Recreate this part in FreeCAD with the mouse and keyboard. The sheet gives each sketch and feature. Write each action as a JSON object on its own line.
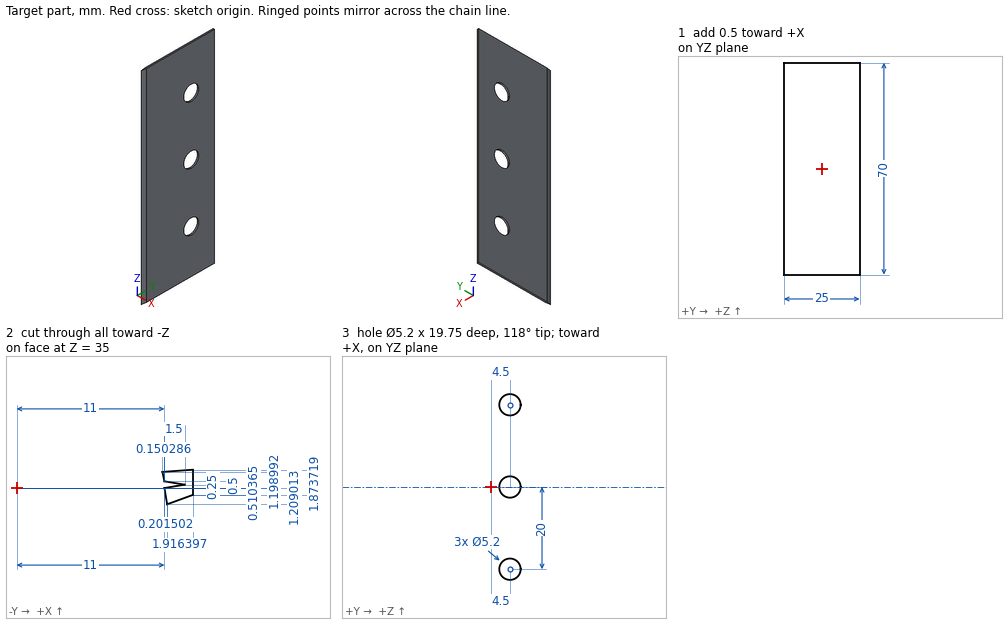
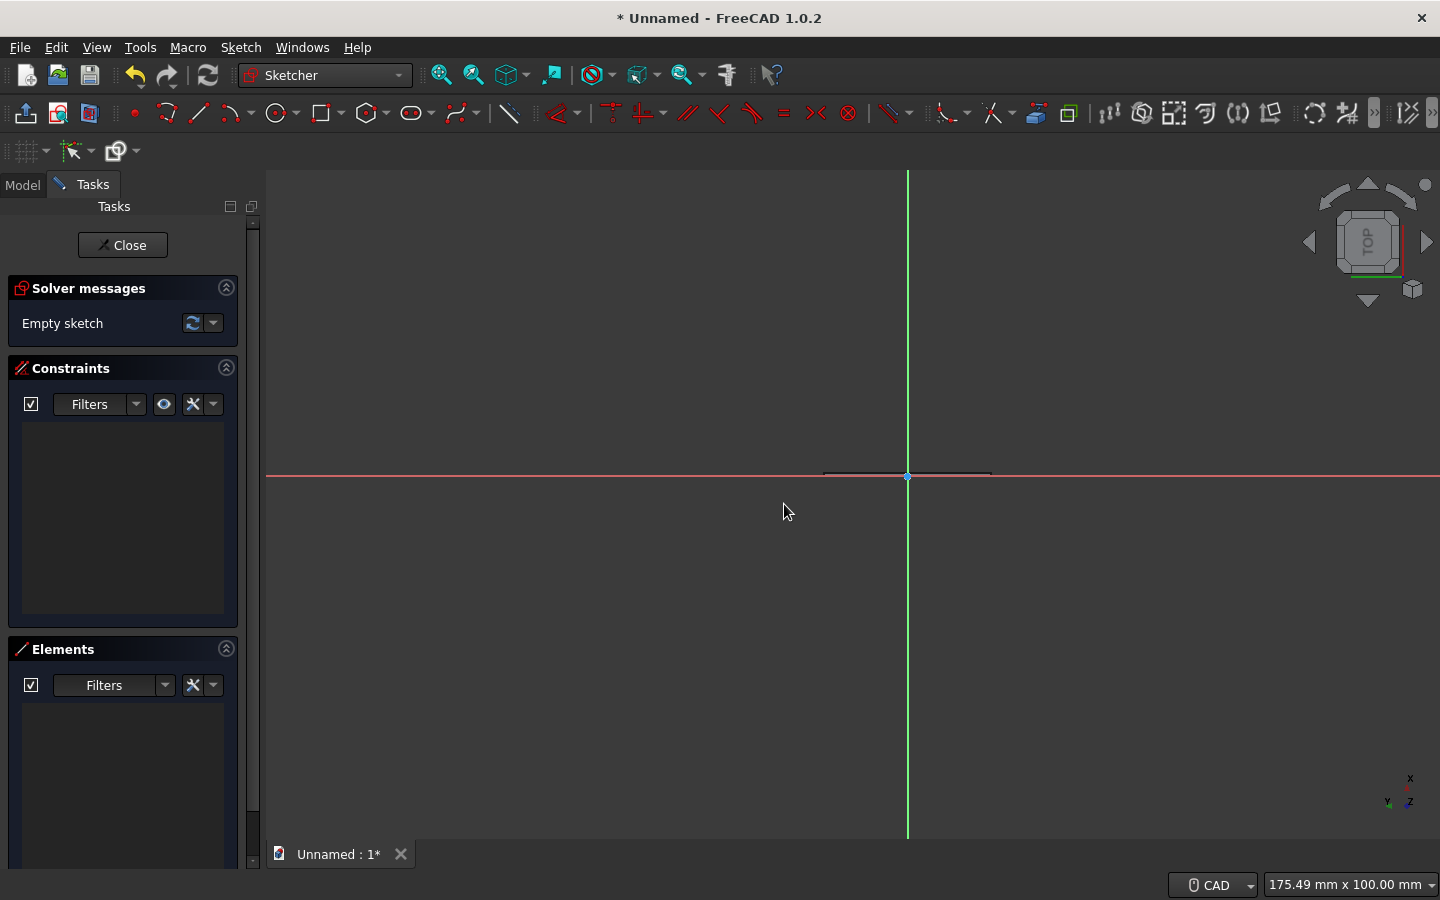
{"action": "scroll", "coordinate": [998, 474], "scroll_direction": "up", "scroll_amount": 15}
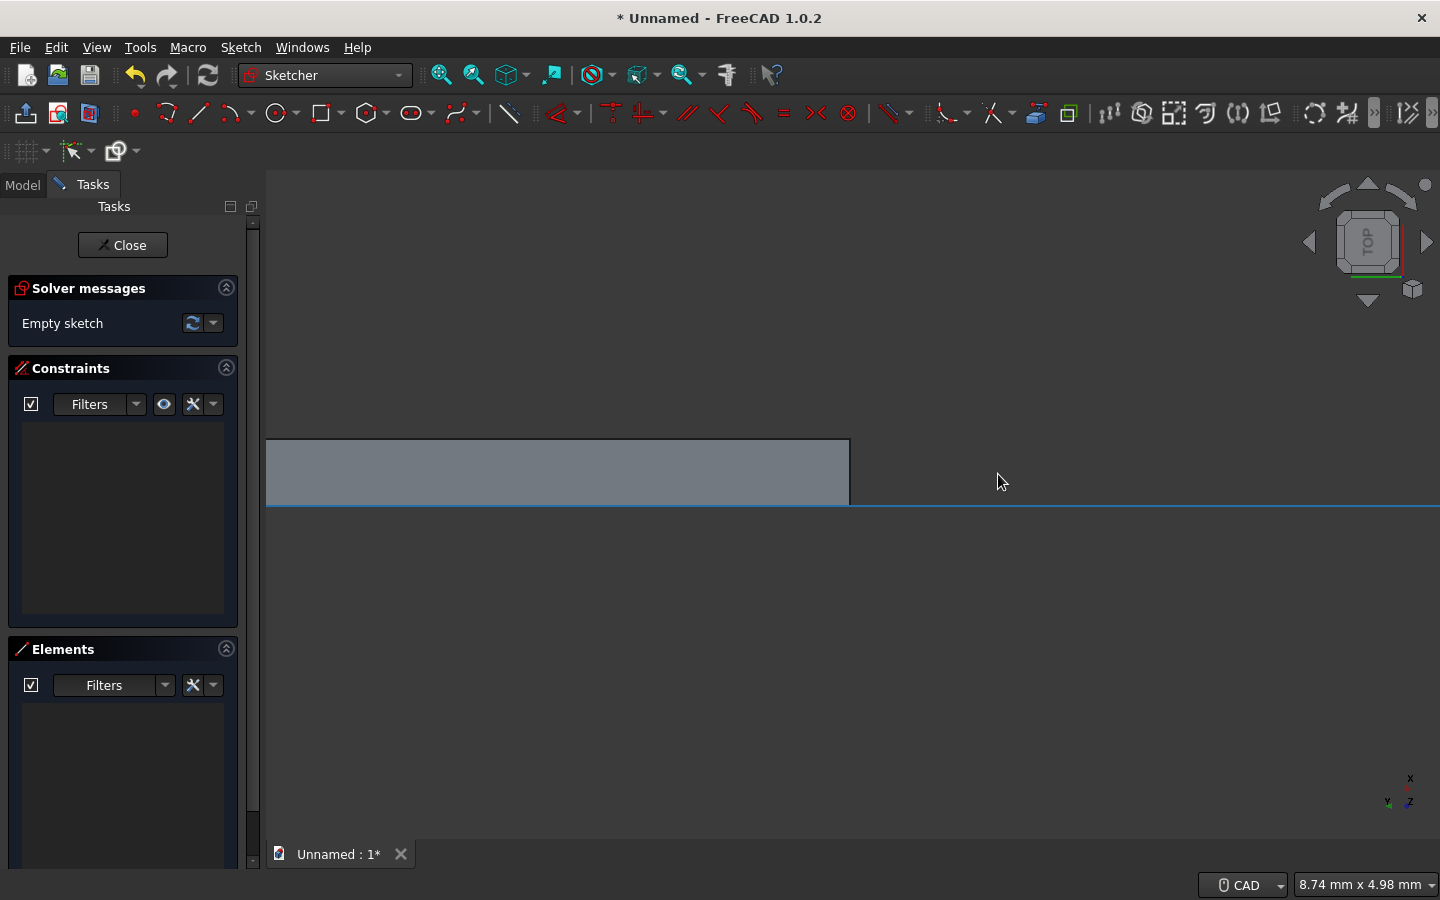
{"action": "left_click", "coordinate": [168, 114]}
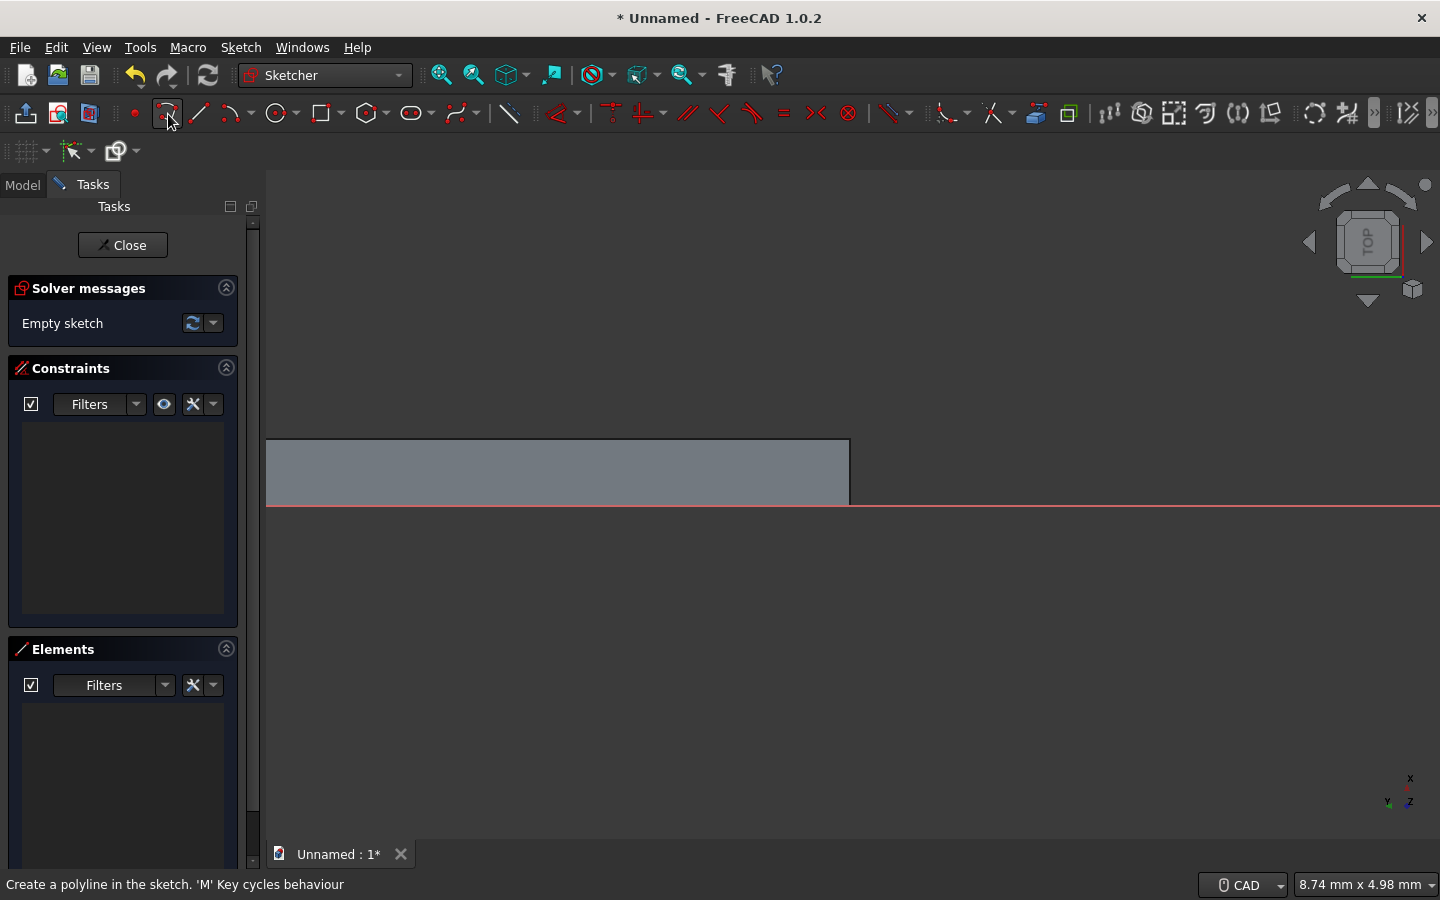
{"action": "left_click", "coordinate": [629, 345]}
{"action": "left_click", "coordinate": [649, 439]}
{"action": "left_click", "coordinate": [850, 473]}
{"action": "left_click", "coordinate": [649, 506]}
{"action": "left_click", "coordinate": [676, 669]}
{"action": "left_click", "coordinate": [933, 575]}
{"action": "left_click", "coordinate": [933, 323]}
{"action": "left_click", "coordinate": [629, 346]}
{"action": "key", "text": "Escape"}
{"action": "key", "text": "Escape"}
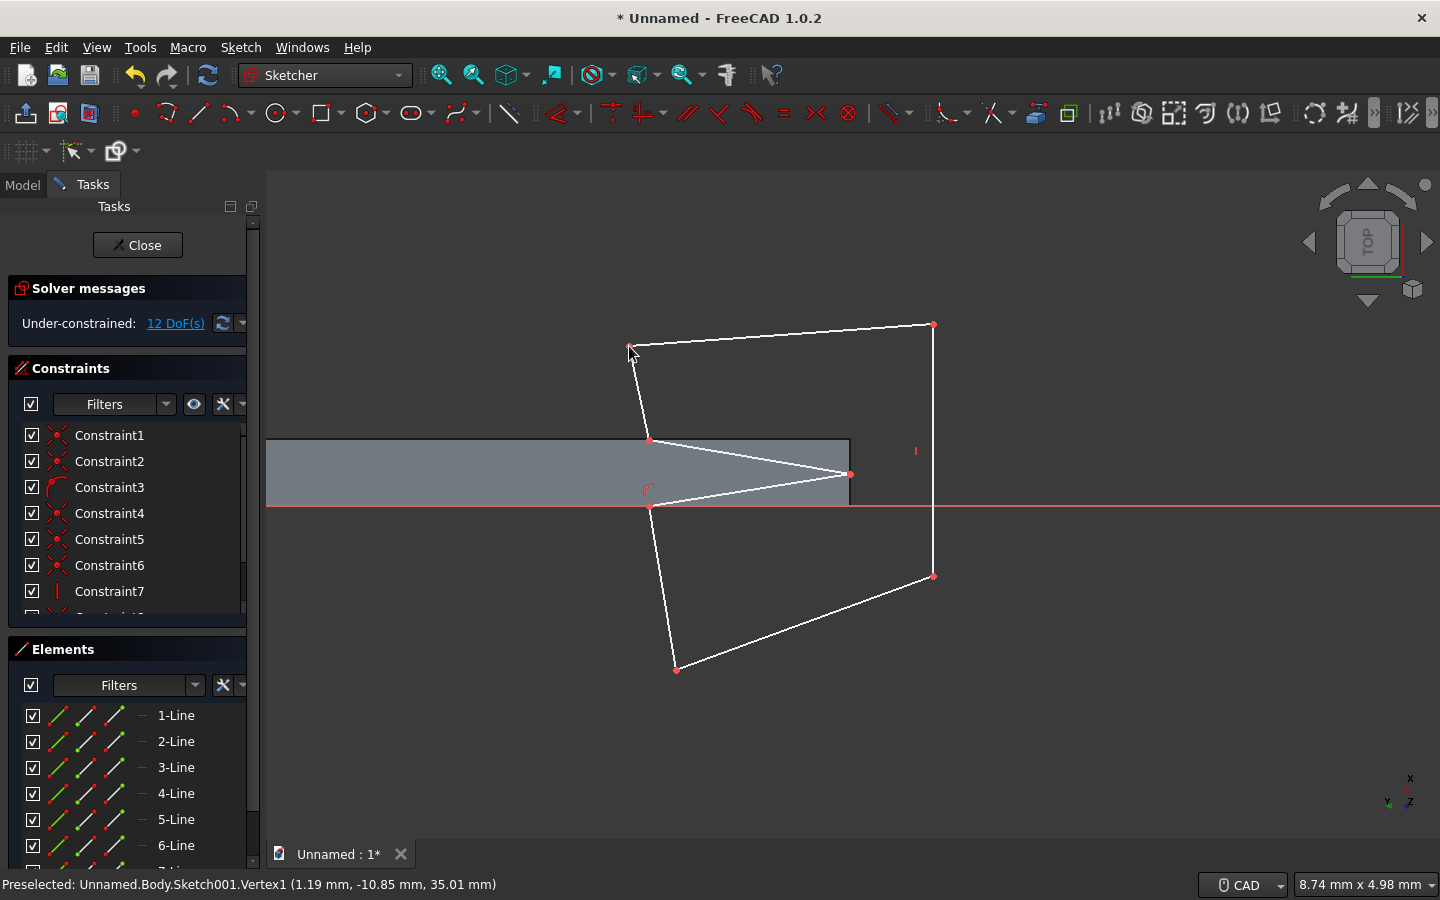
{"action": "key", "text": "d"}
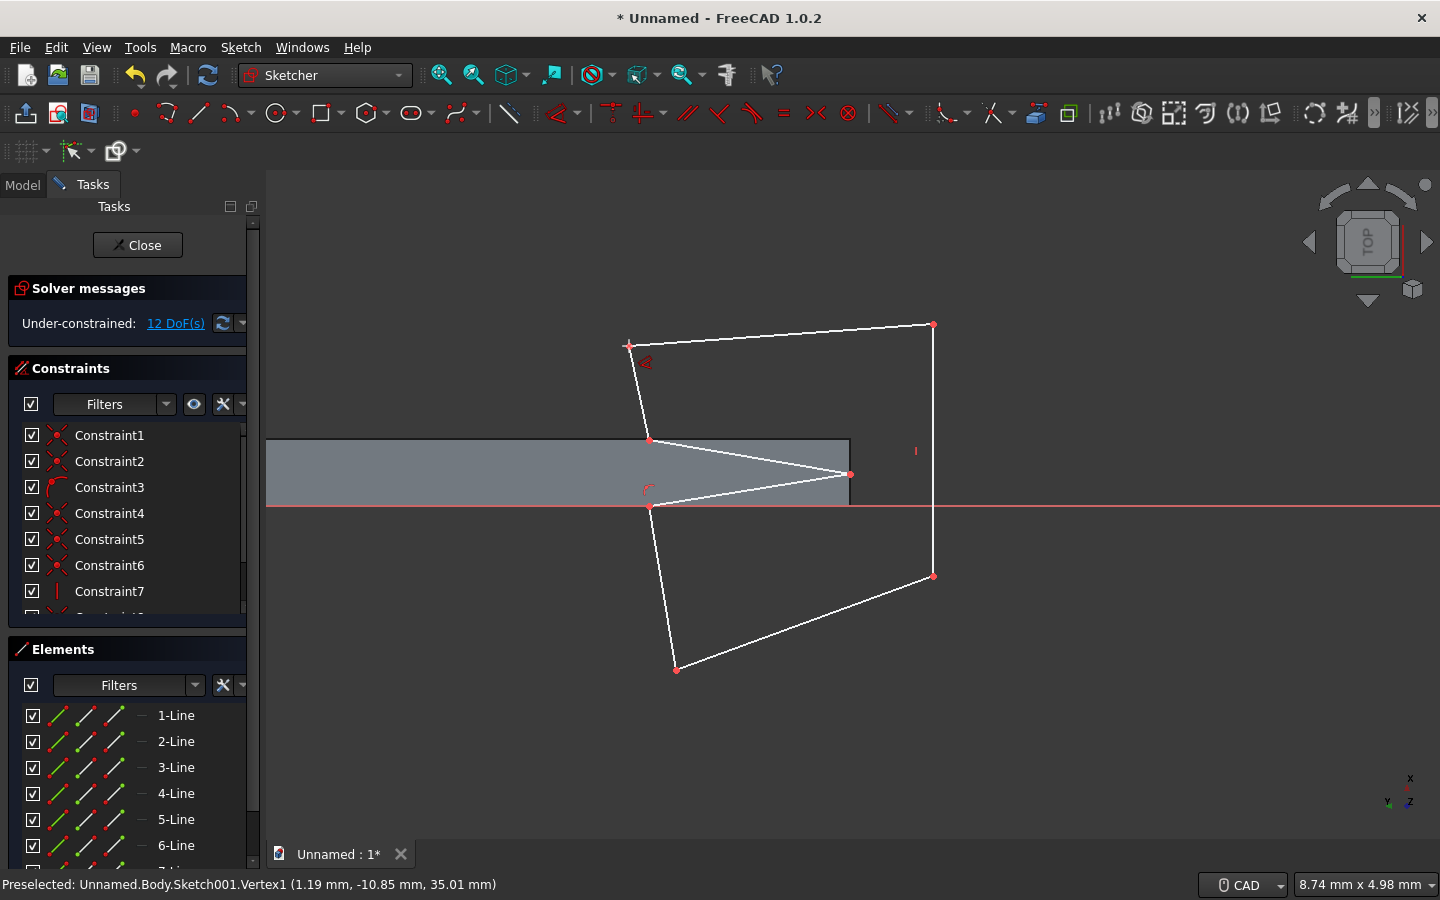
{"action": "left_click", "coordinate": [649, 440]}
{"action": "left_click", "coordinate": [472, 406]}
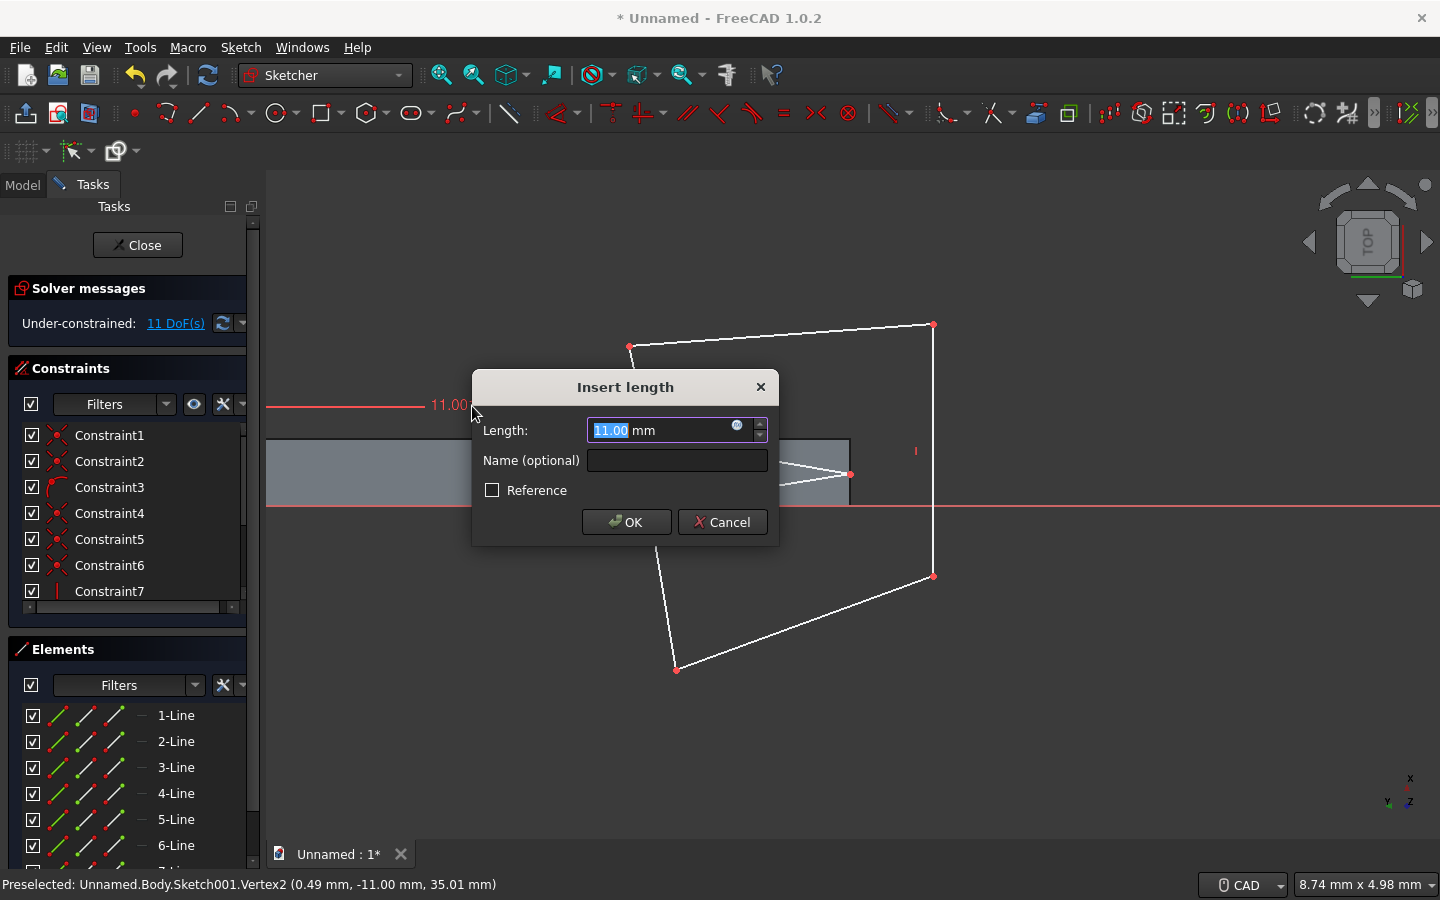
{"action": "type", "text": "11"}
{"action": "key", "text": "Return"}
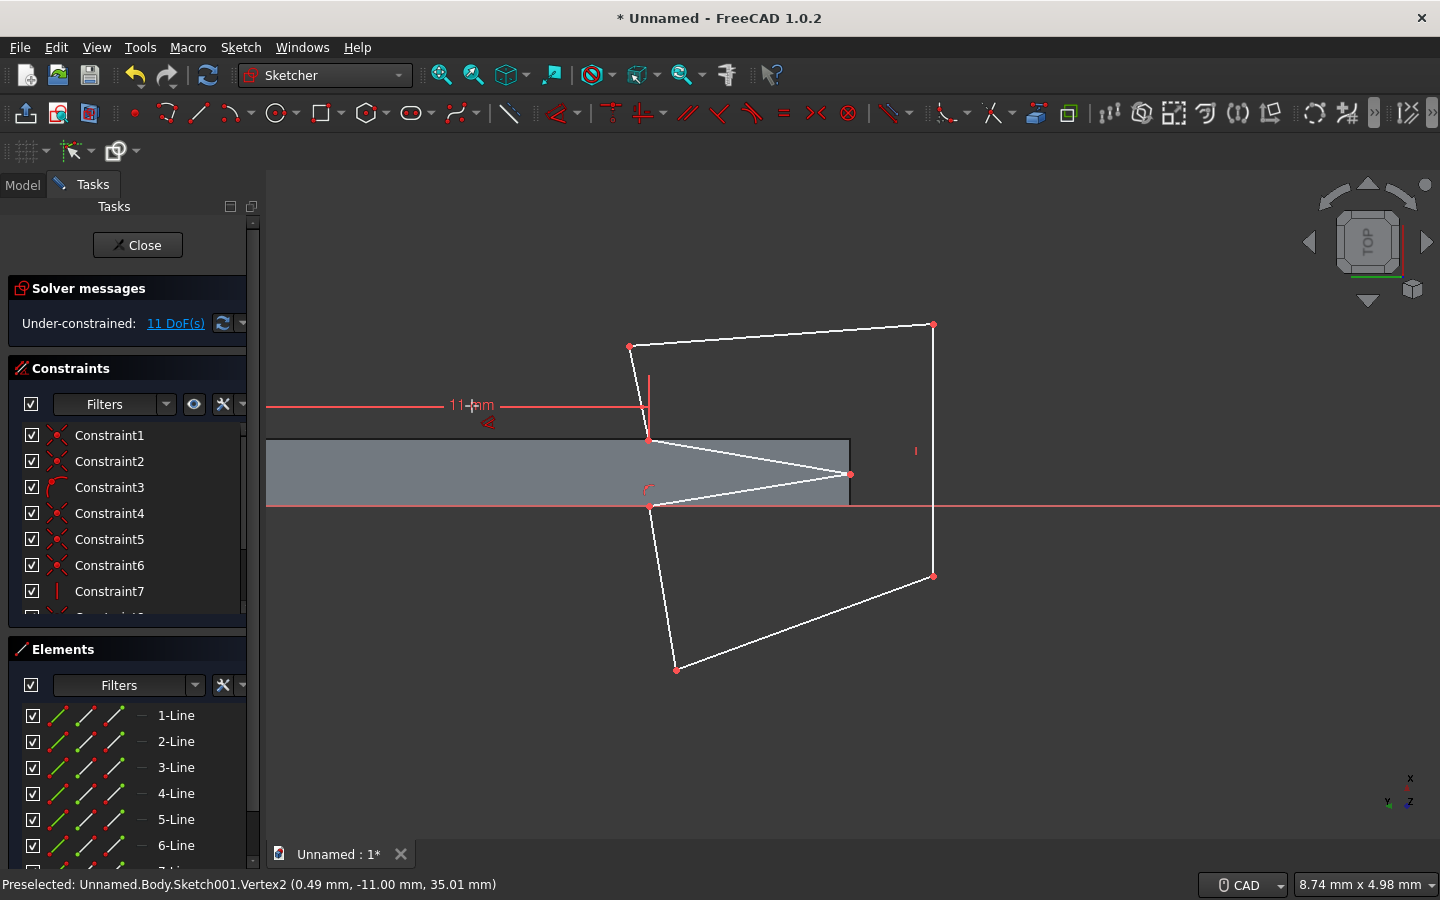
{"action": "left_click", "coordinate": [649, 506]}
{"action": "left_click", "coordinate": [472, 540]}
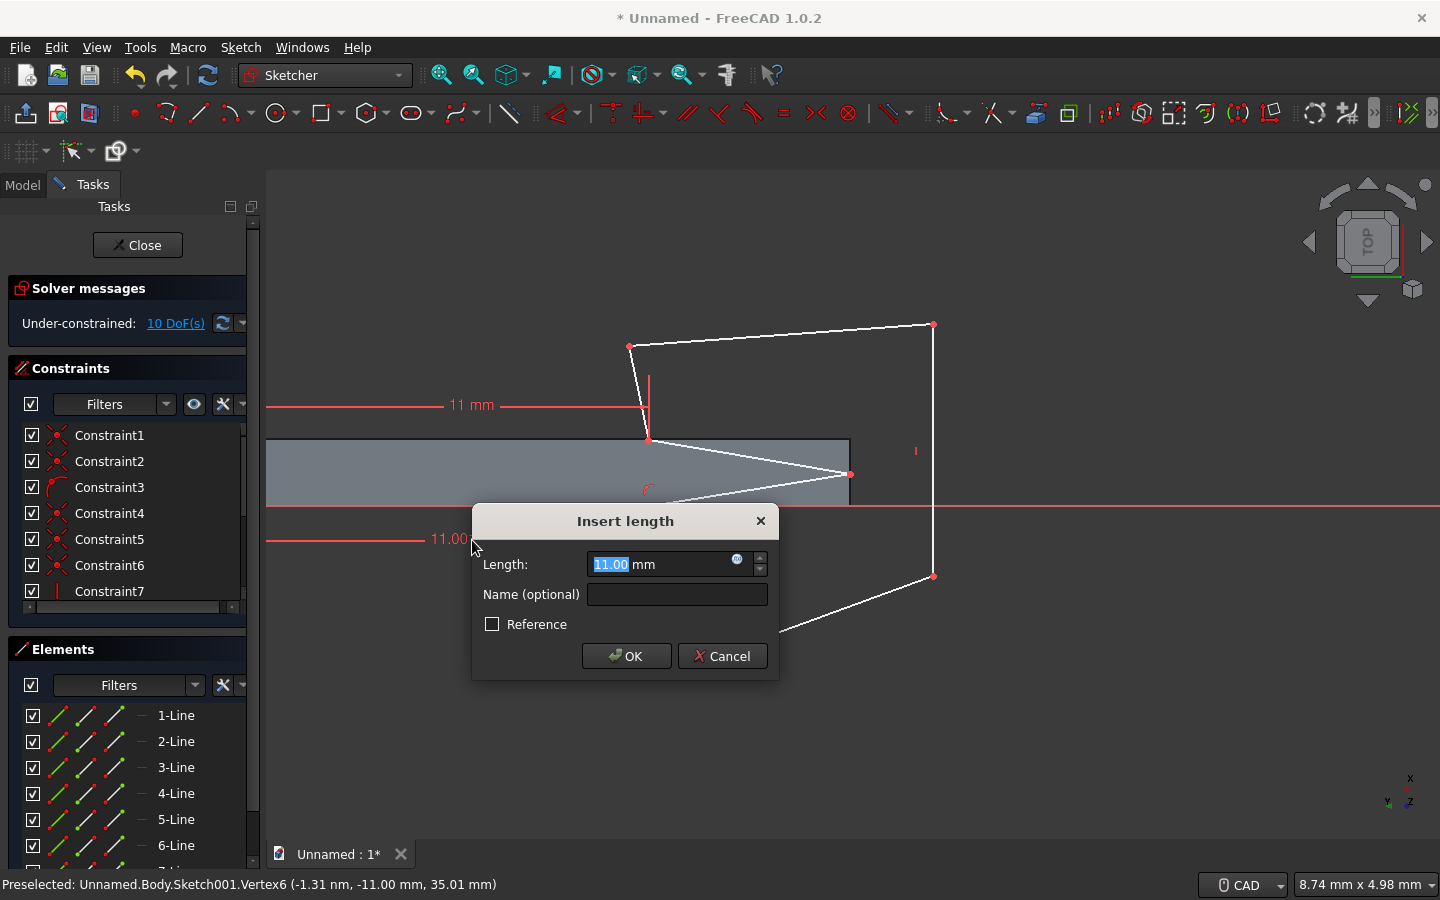
{"action": "type", "text": "11"}
{"action": "key", "text": "Return"}